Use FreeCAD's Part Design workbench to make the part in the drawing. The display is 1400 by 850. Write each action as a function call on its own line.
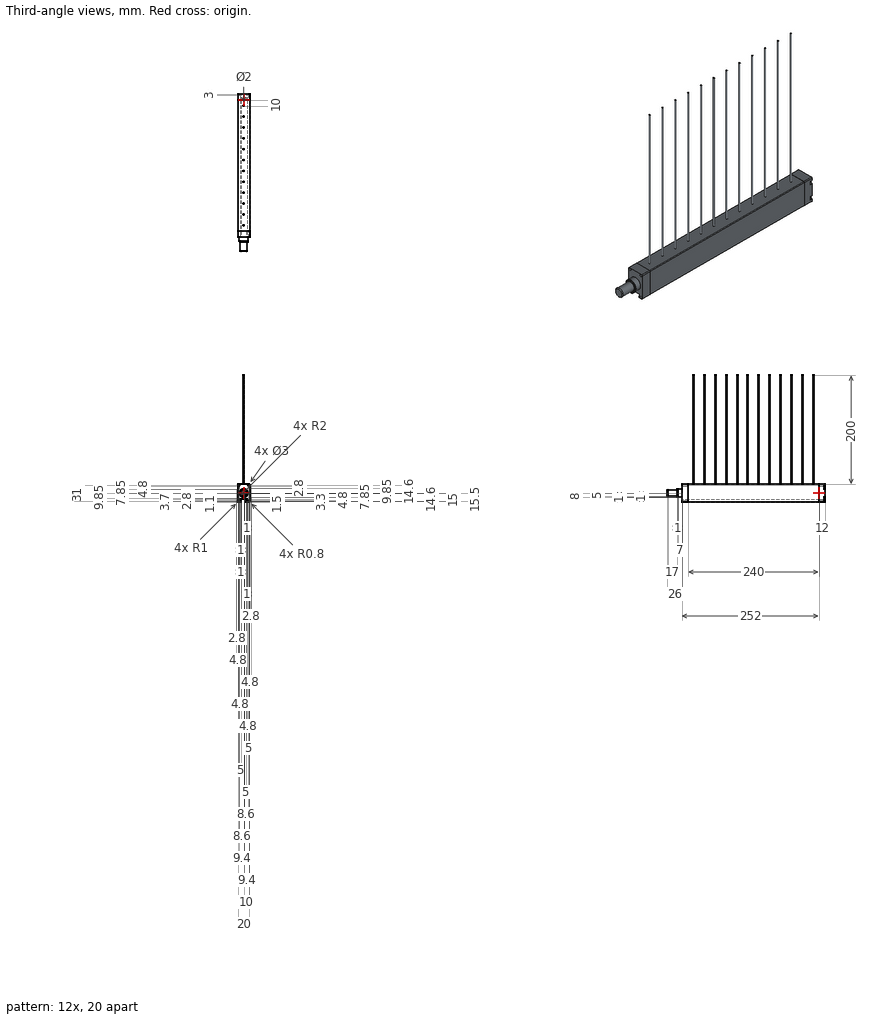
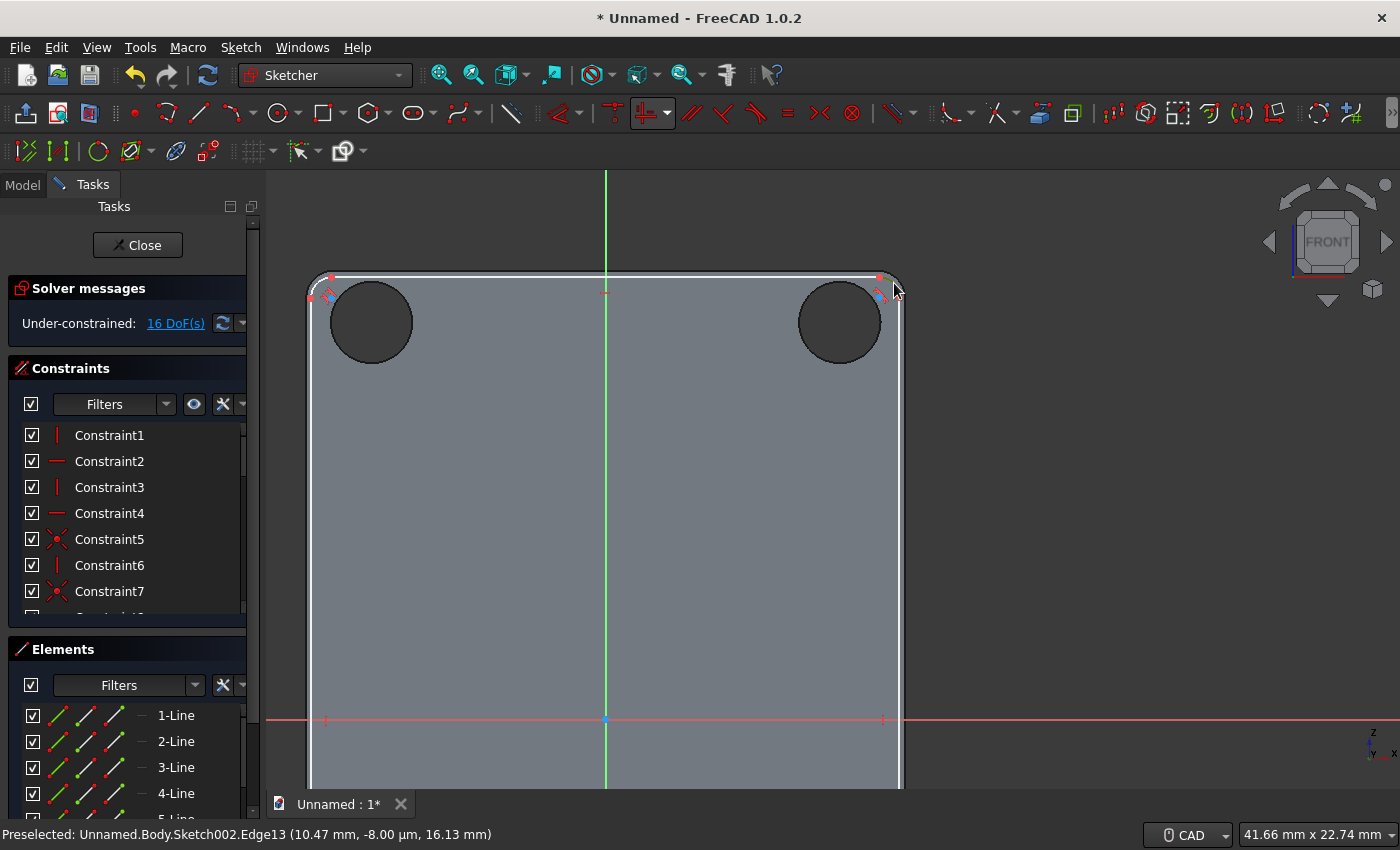
scroll(322, 280, up, 2)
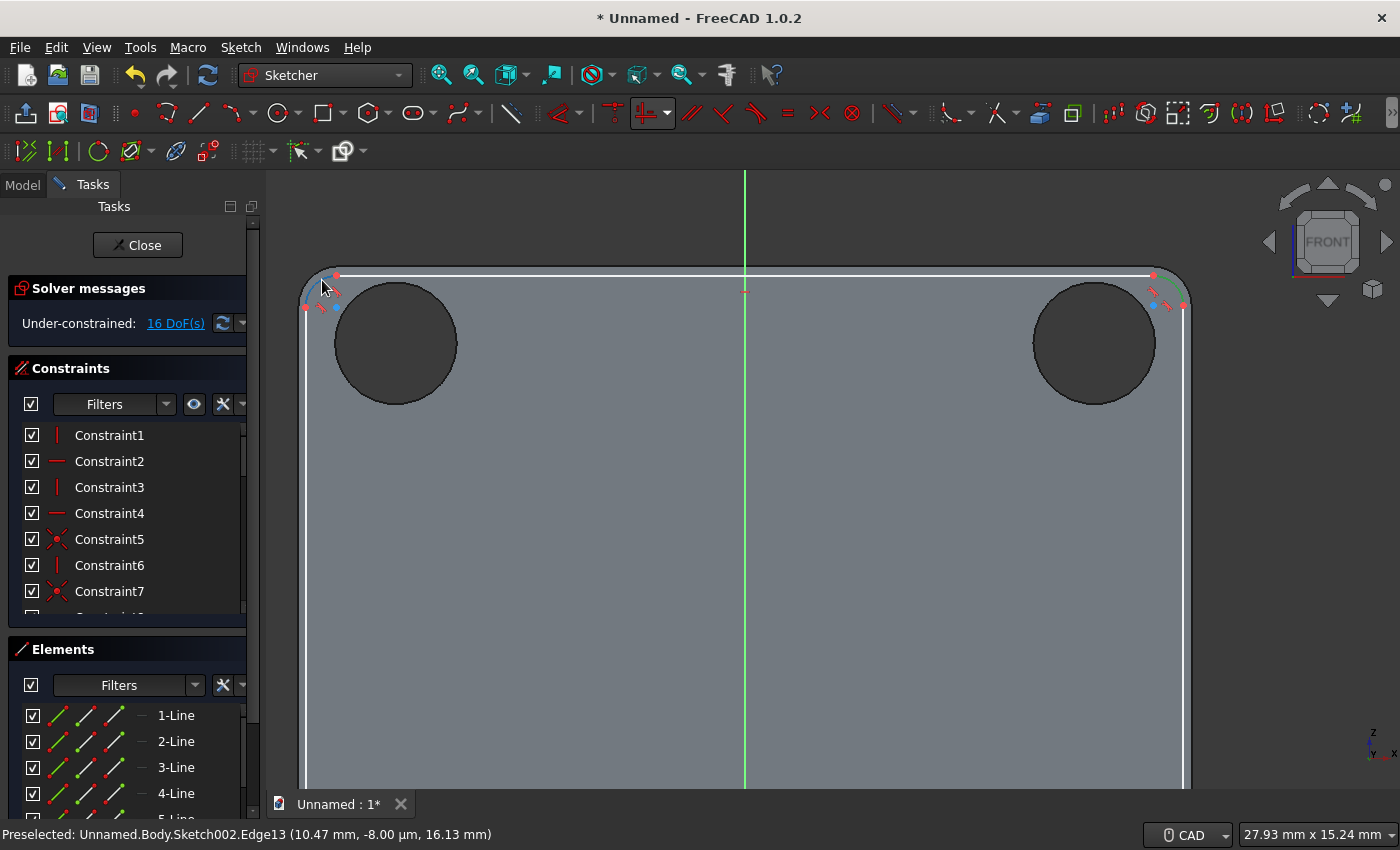
click(323, 279)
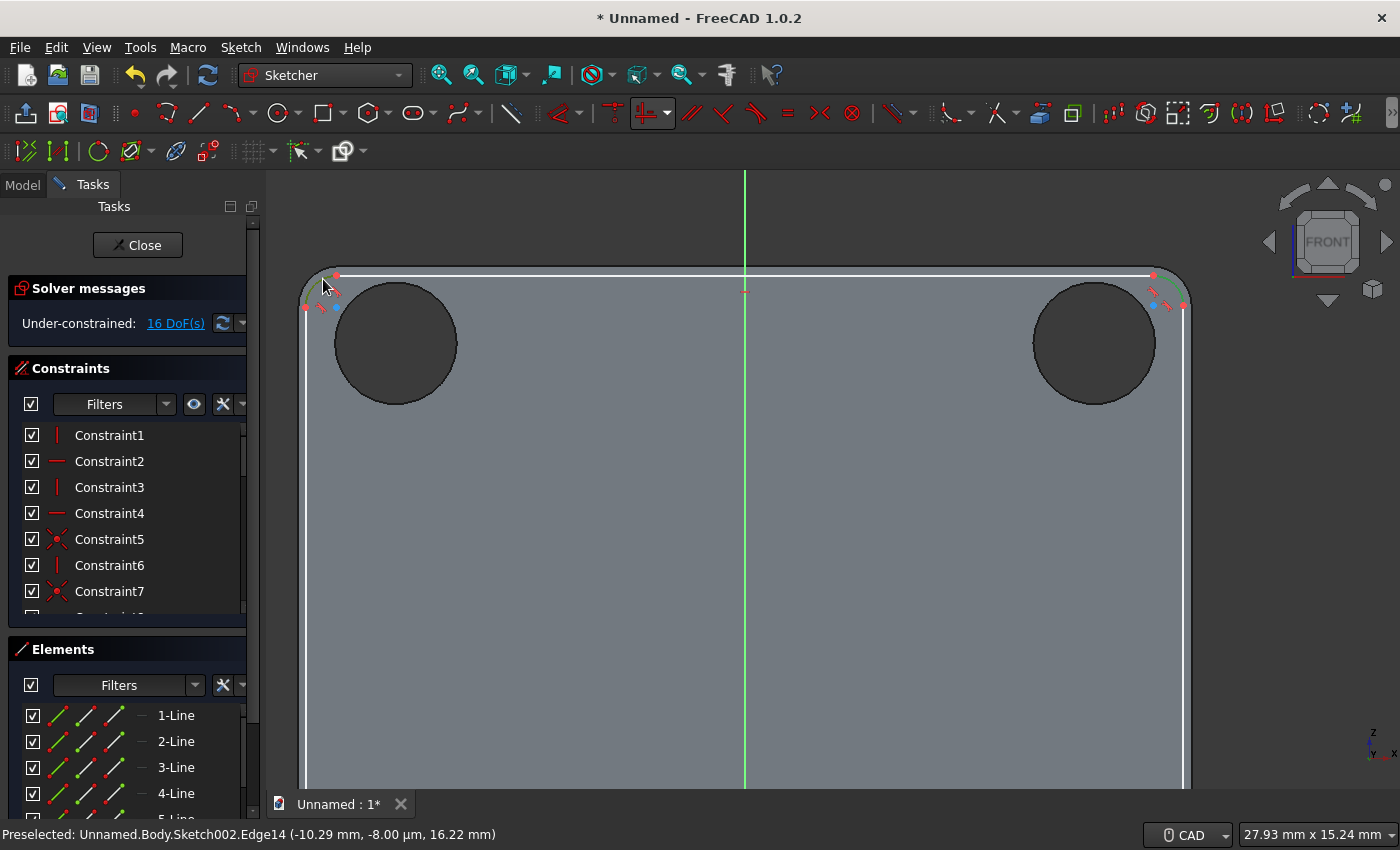
scroll(773, 283, down, 6)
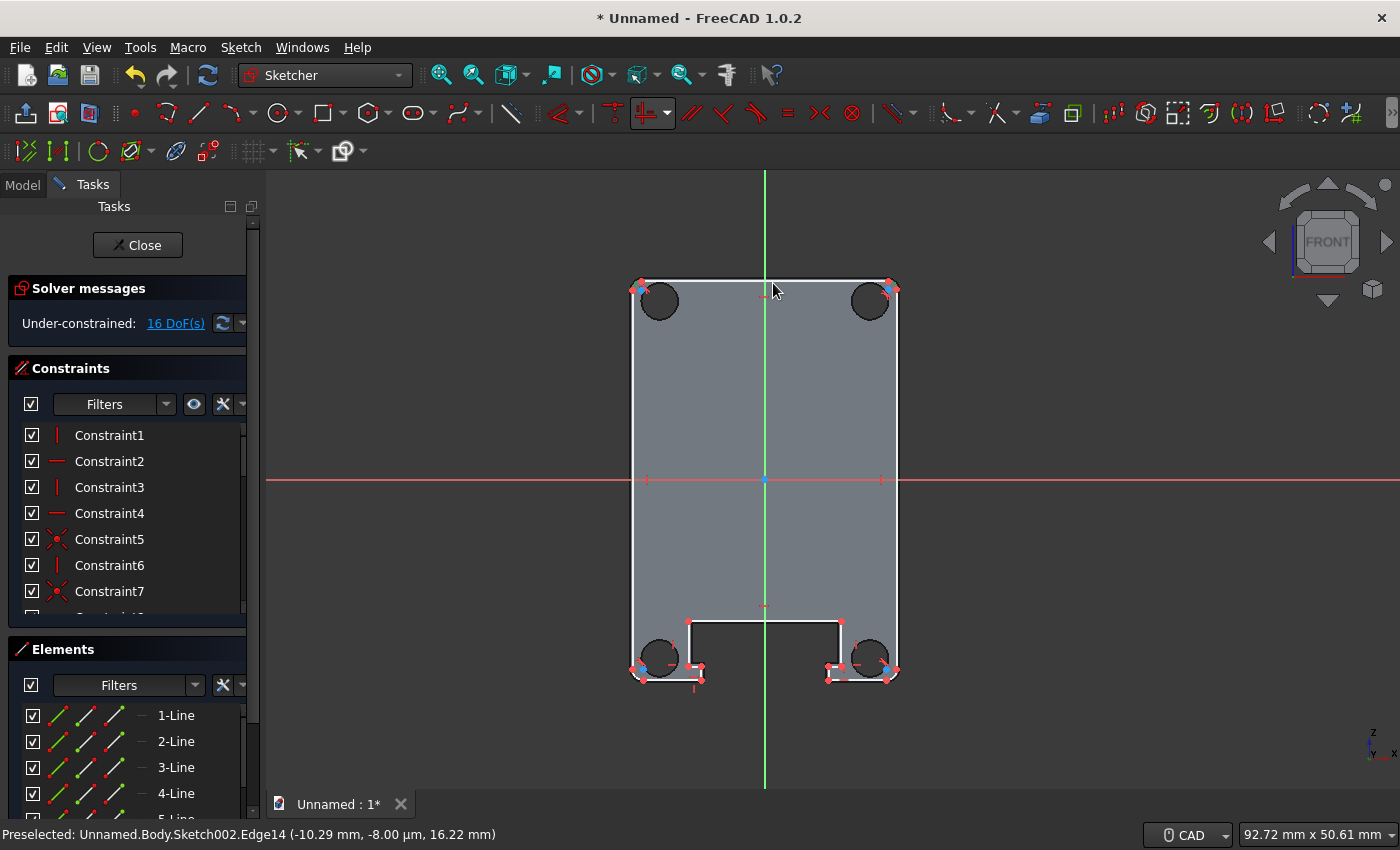
scroll(634, 674, up, 6)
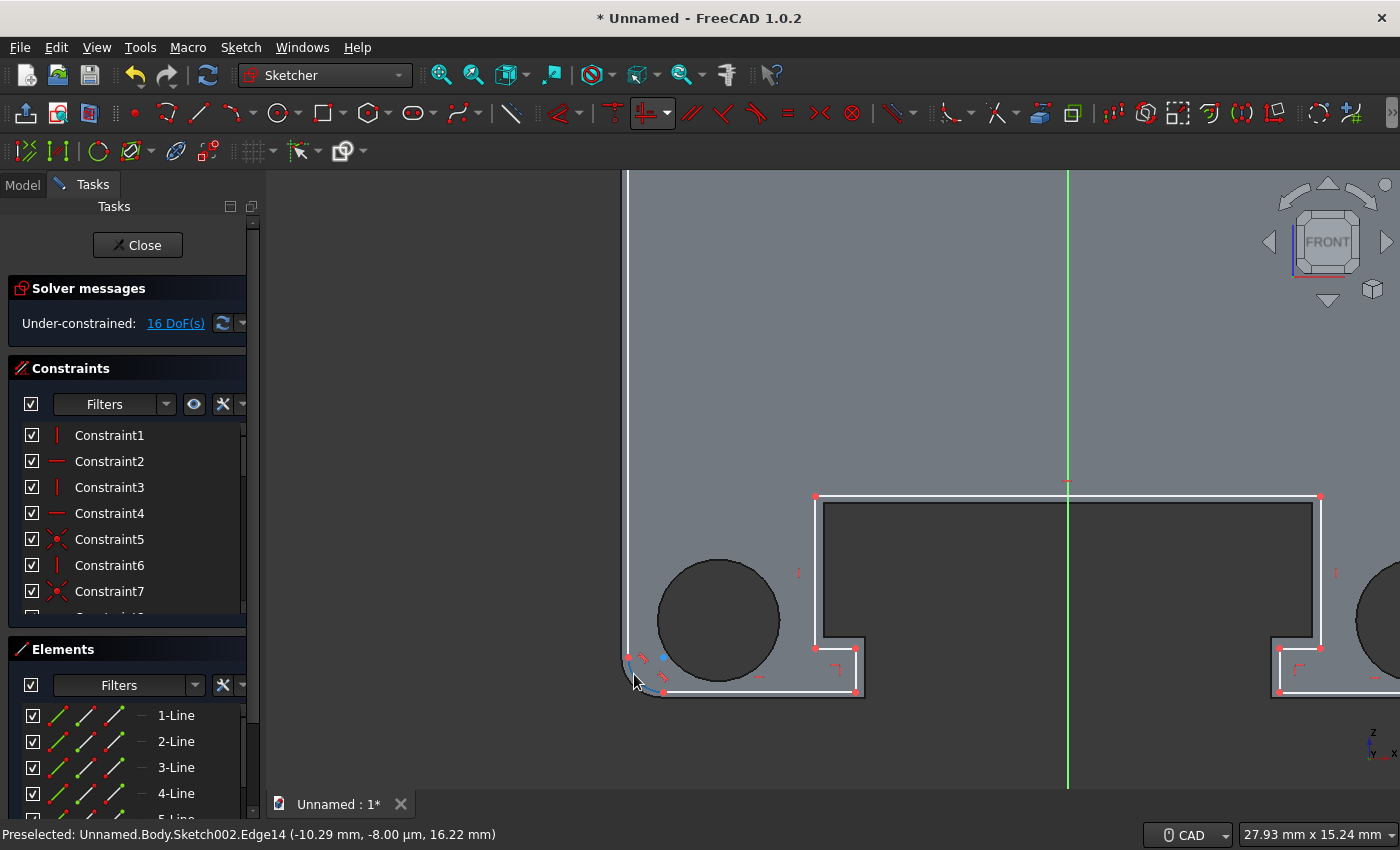
click(632, 673)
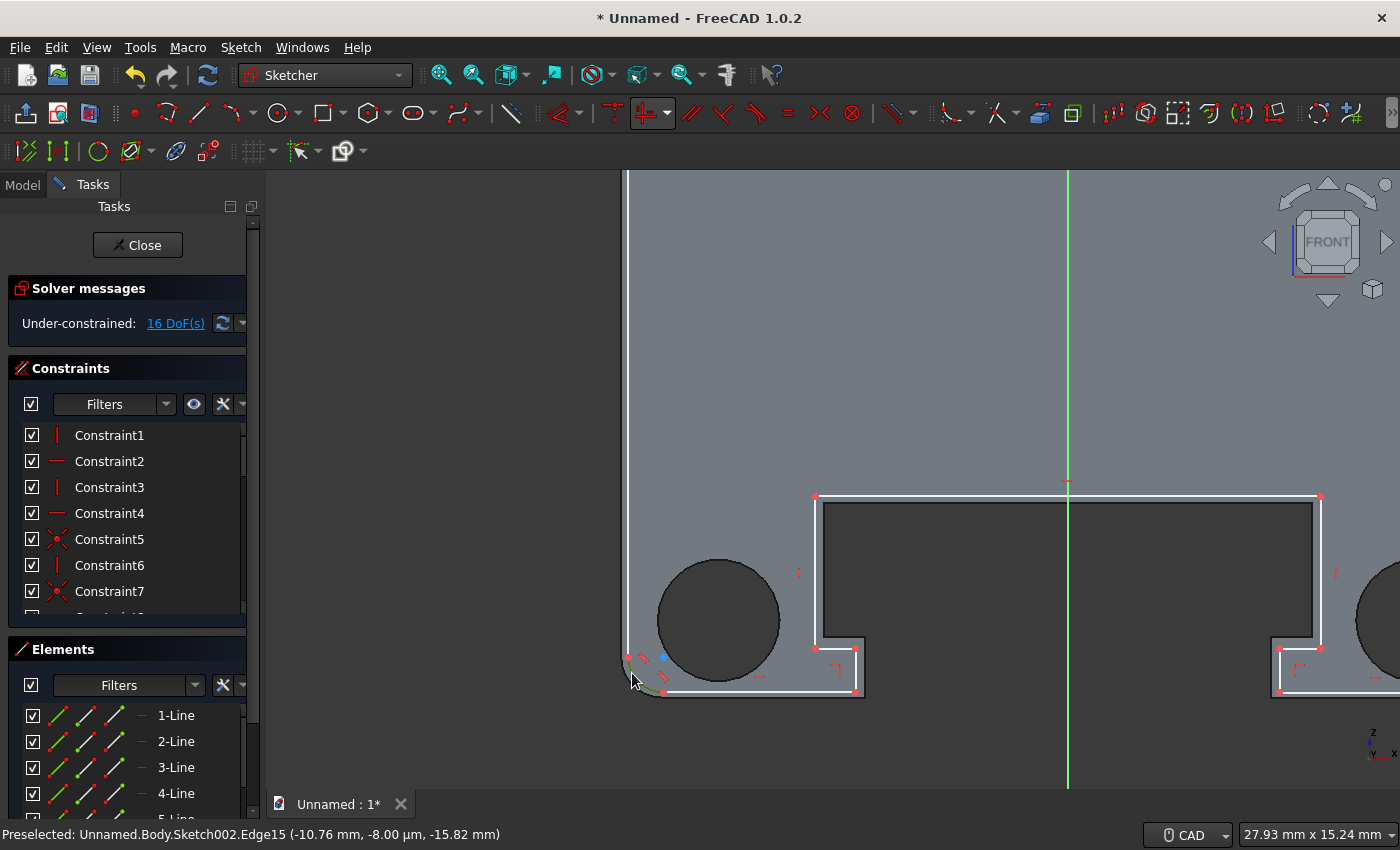
scroll(634, 674, down, 6)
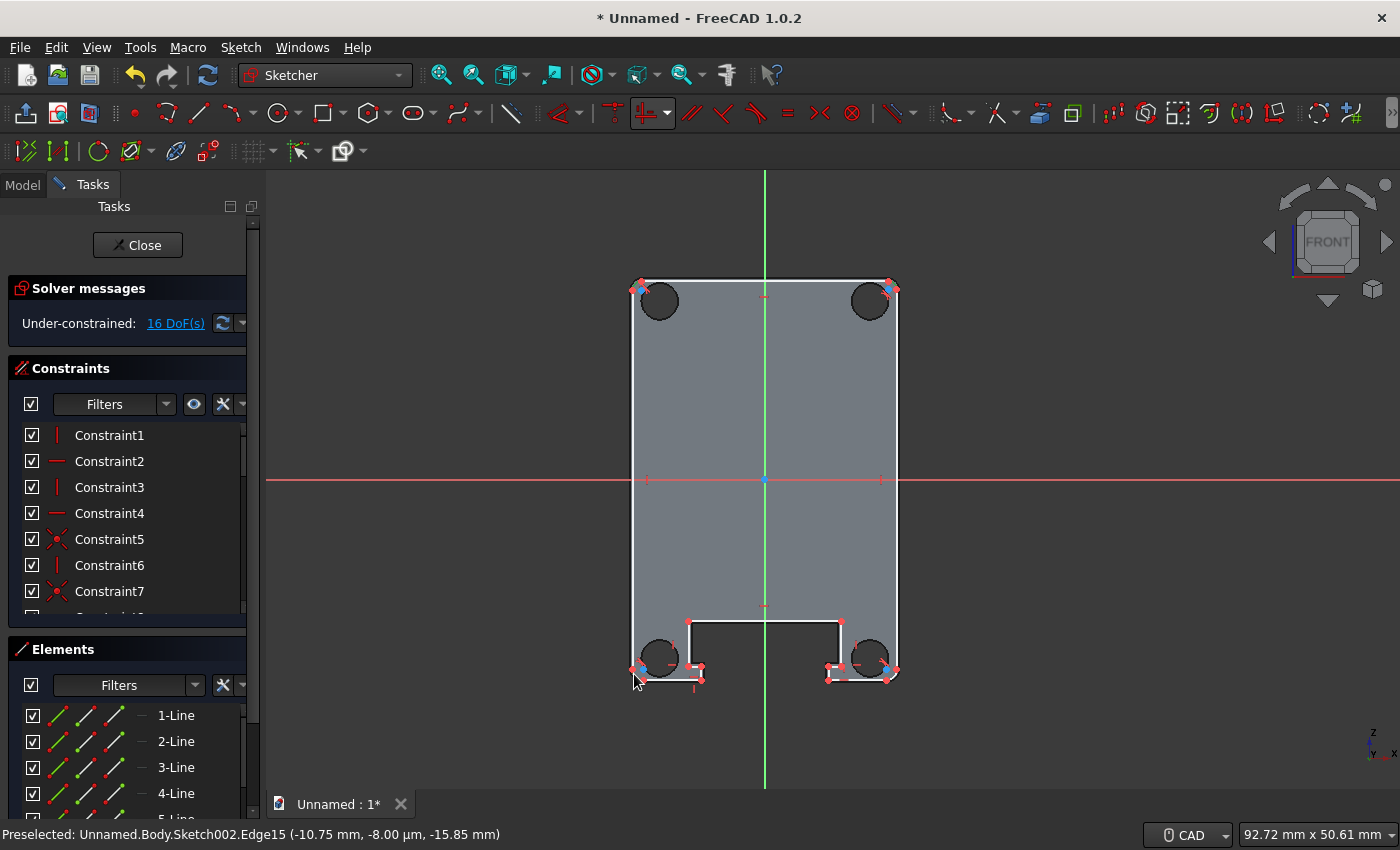
scroll(891, 679, up, 6)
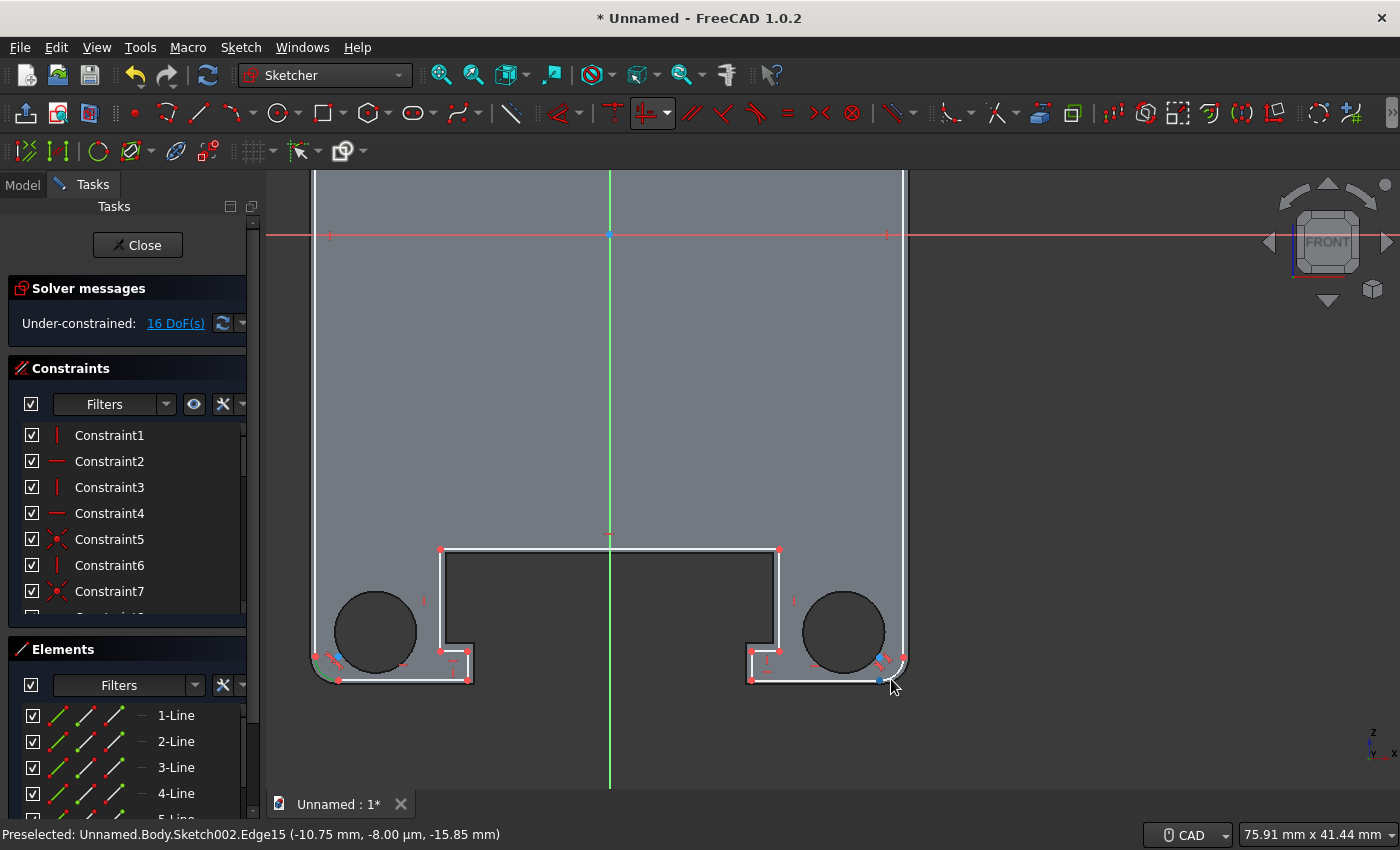
click(890, 677)